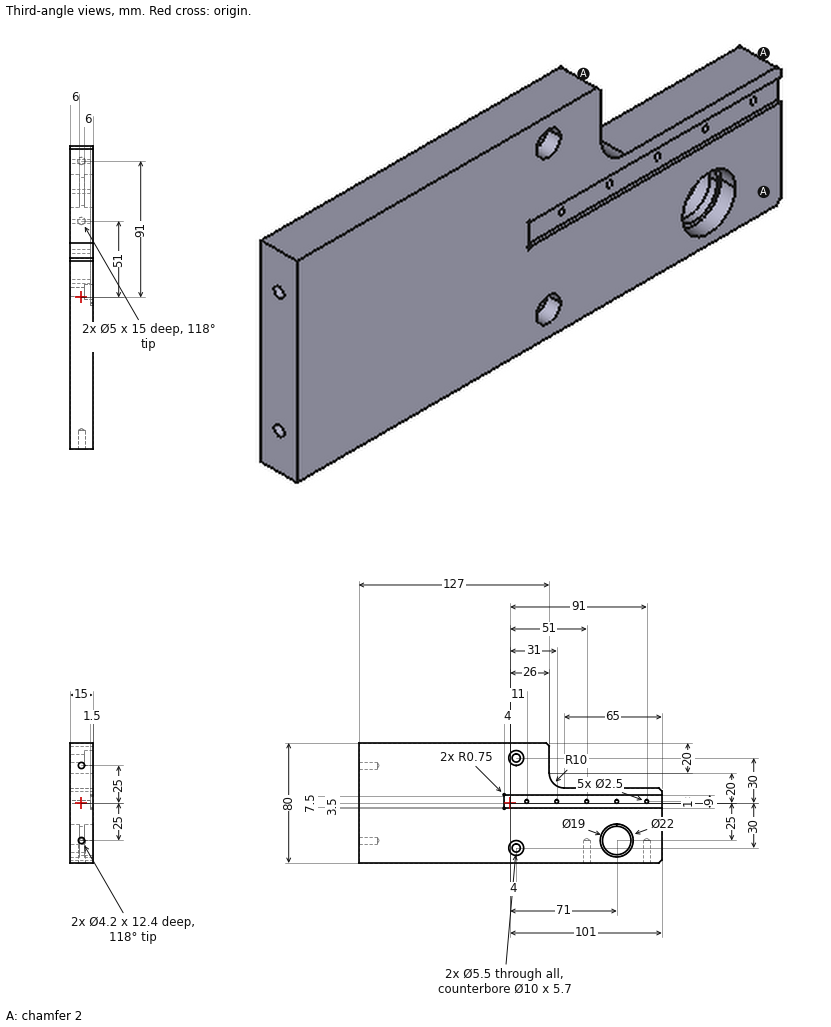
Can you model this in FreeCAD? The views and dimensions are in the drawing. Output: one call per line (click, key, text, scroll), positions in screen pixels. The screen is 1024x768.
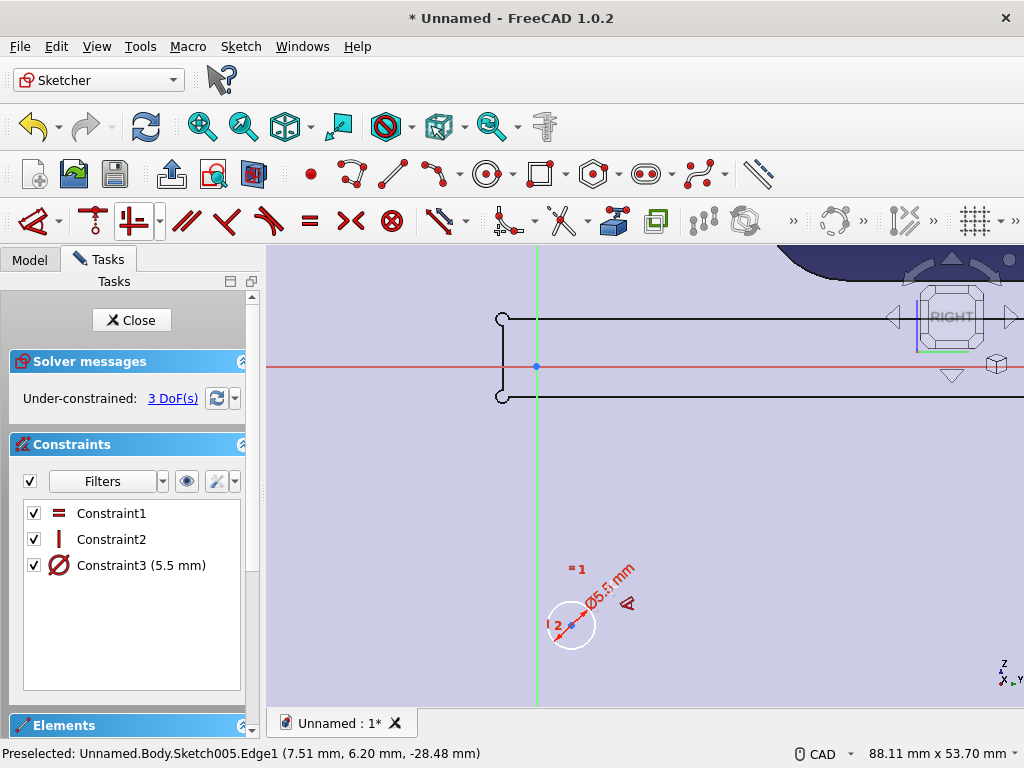
click(571, 625)
click(554, 659)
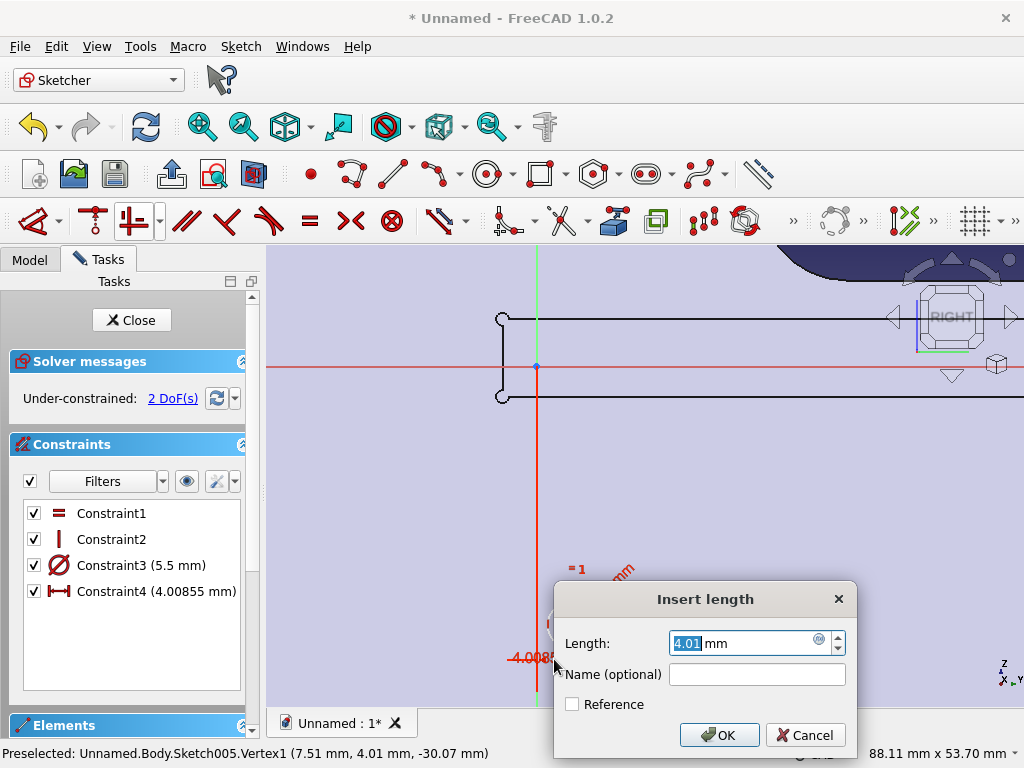
text(4)
key(Return)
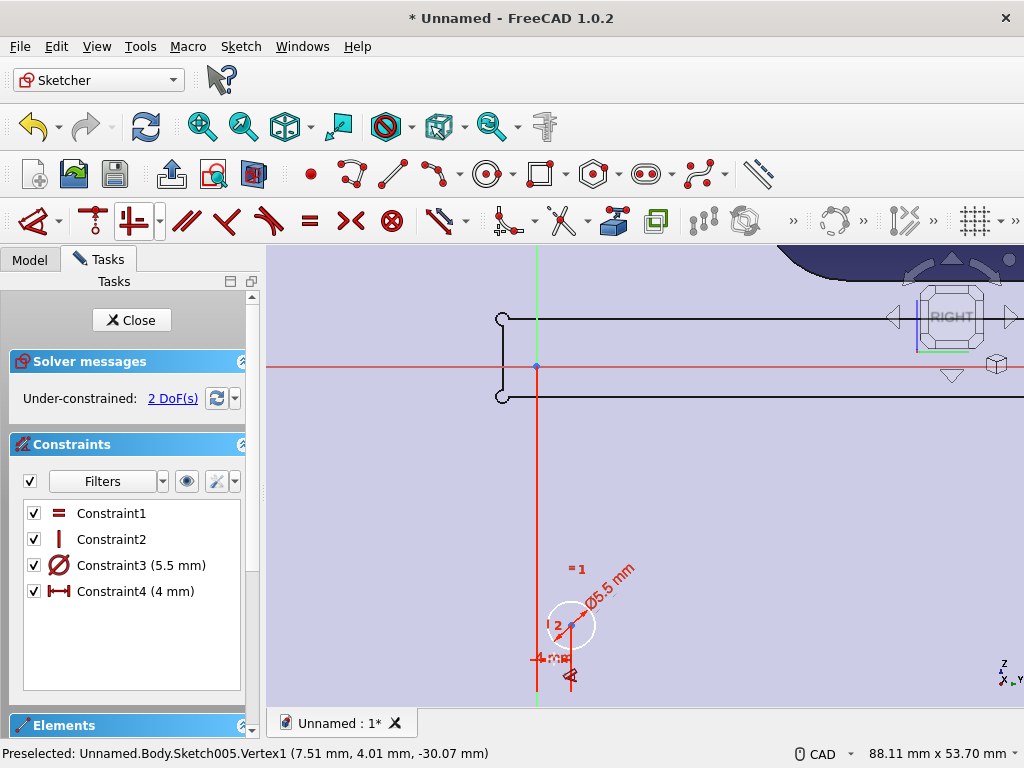
click(571, 625)
click(503, 496)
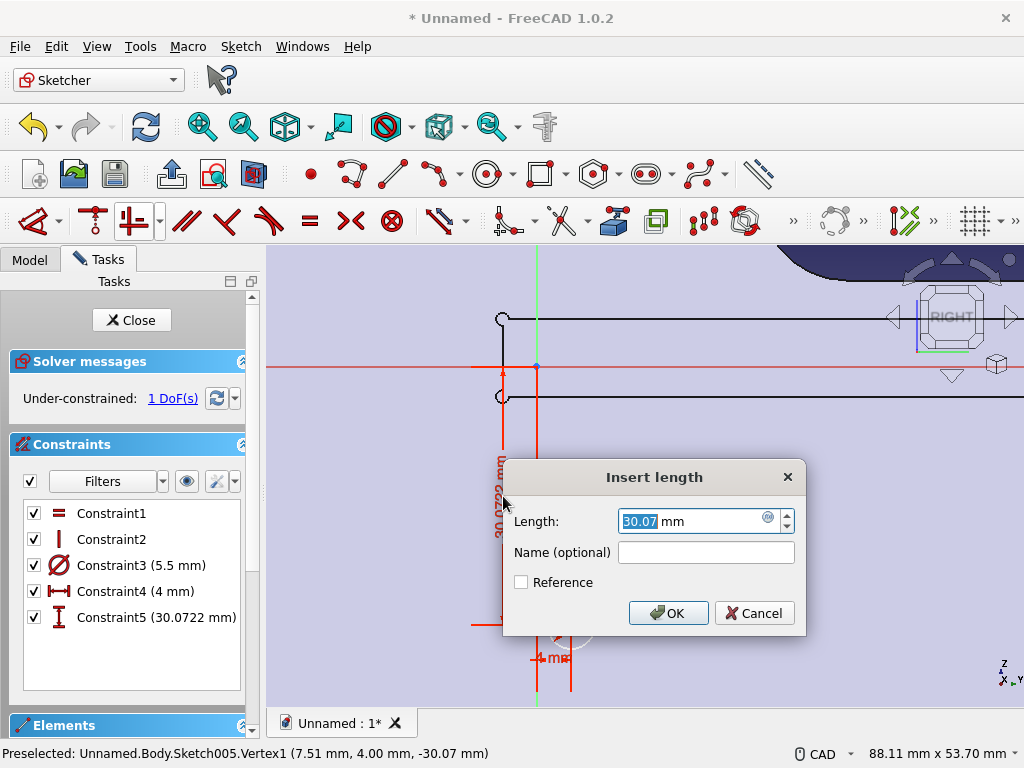
text(30)
key(Return)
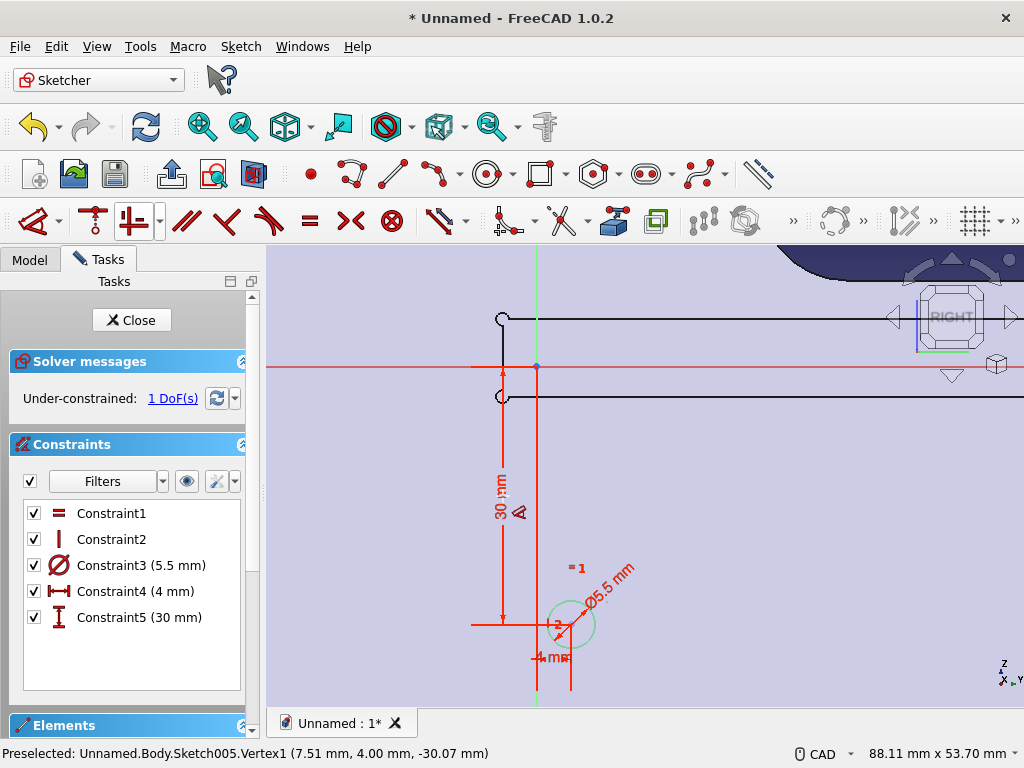
scroll(589, 609, down, 3)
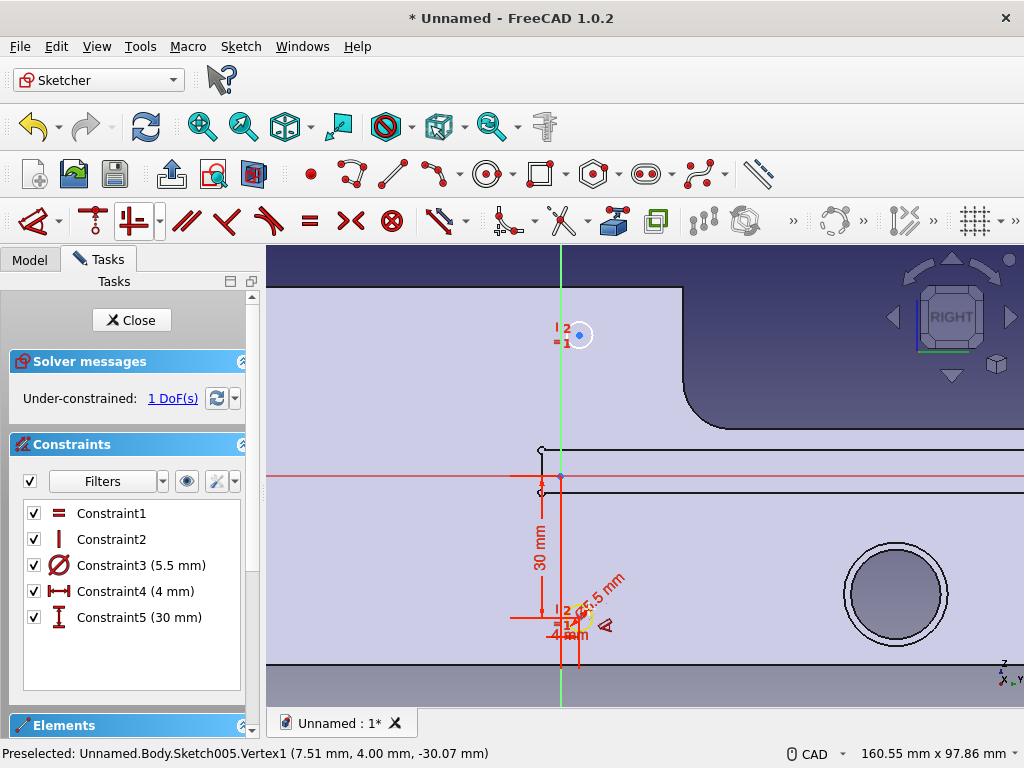
click(580, 335)
click(527, 406)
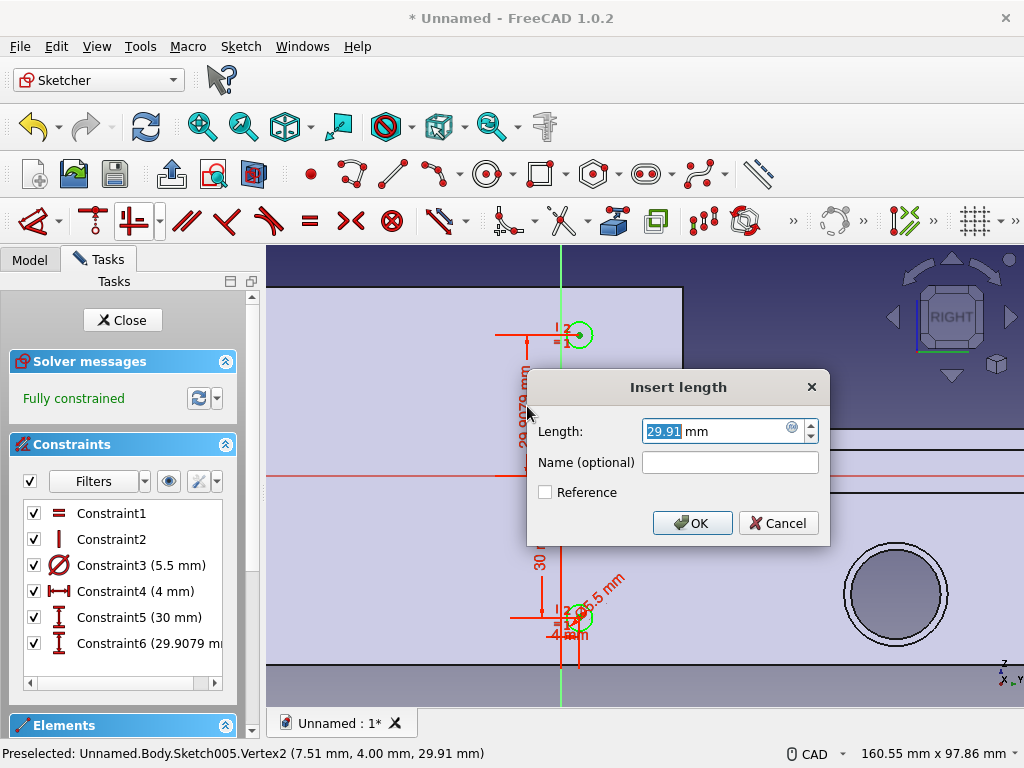
text(30)
key(Return)
key(Escape)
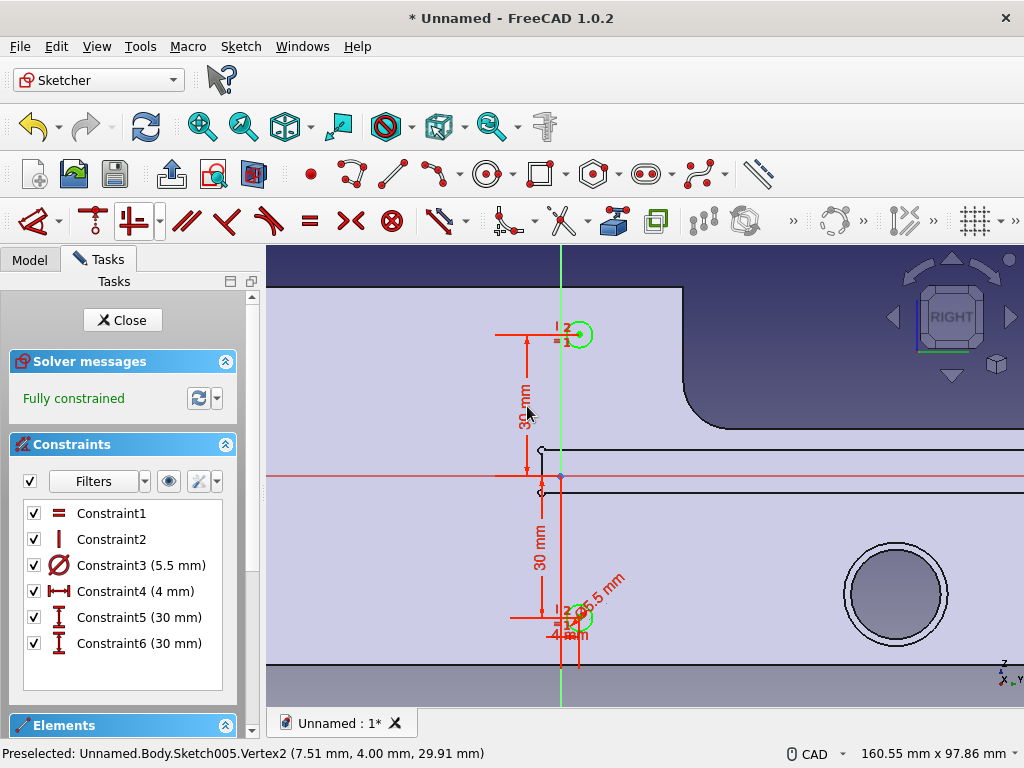
click(123, 320)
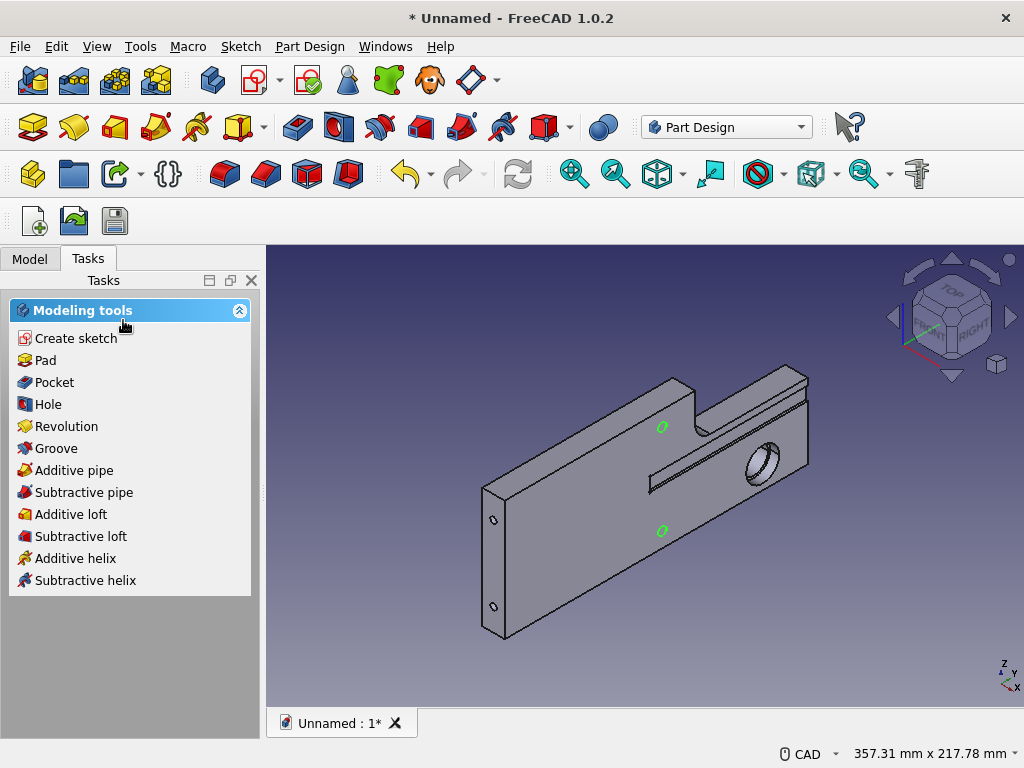
click(339, 128)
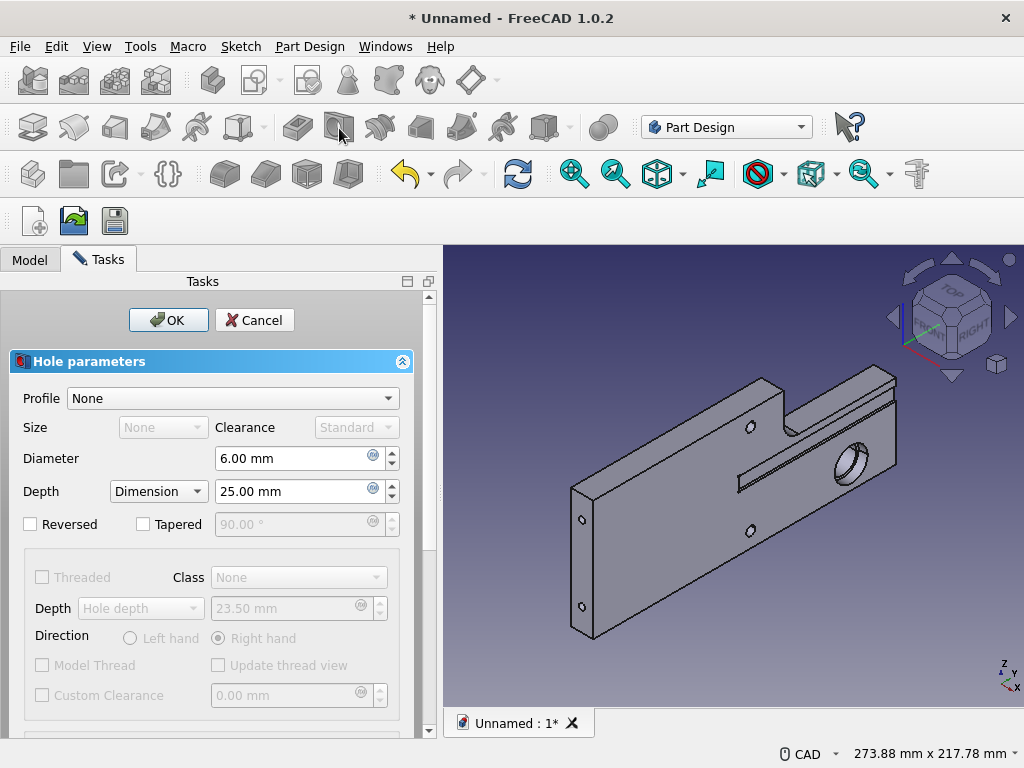
triple_click(300, 458)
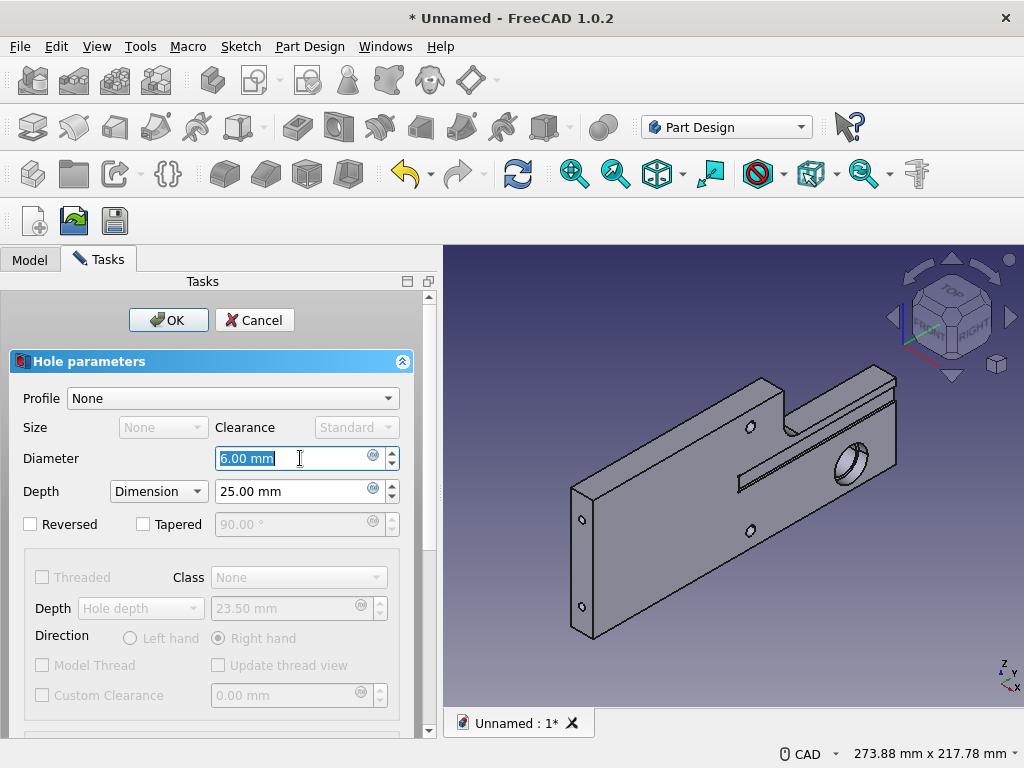
text(5.5)
key(Tab)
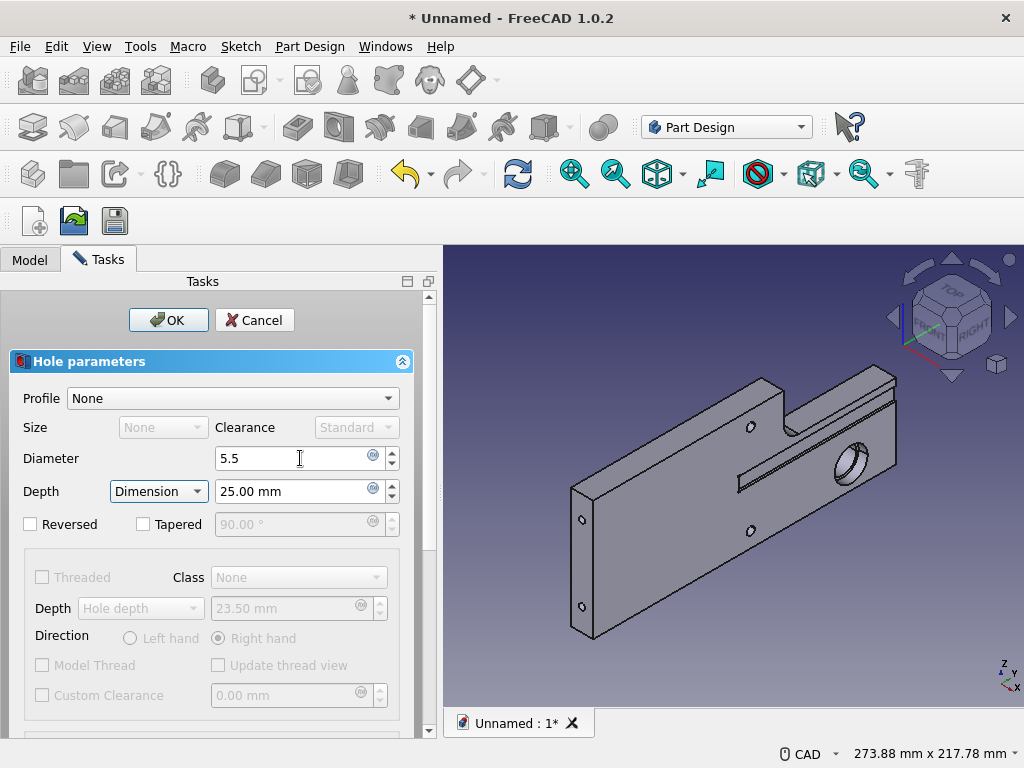
click(160, 492)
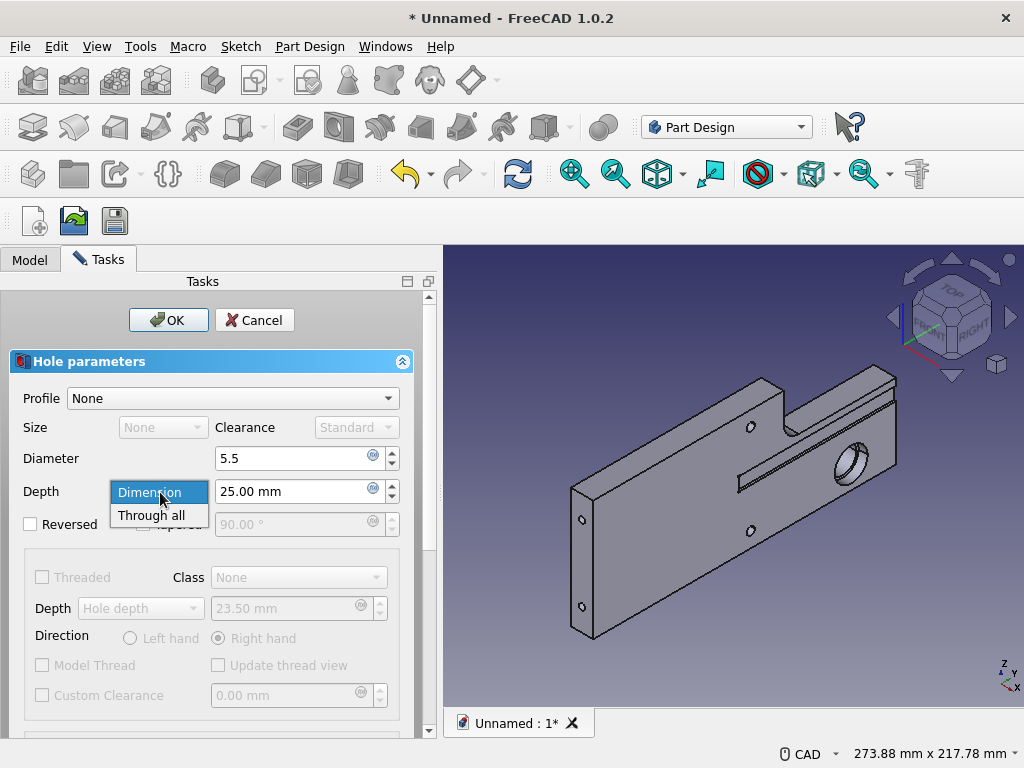
click(158, 516)